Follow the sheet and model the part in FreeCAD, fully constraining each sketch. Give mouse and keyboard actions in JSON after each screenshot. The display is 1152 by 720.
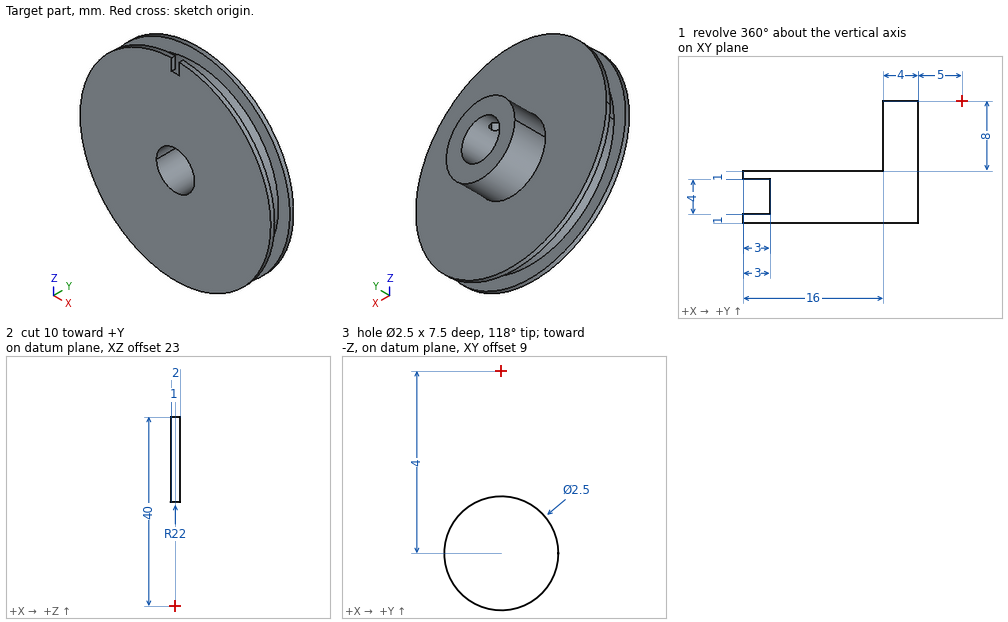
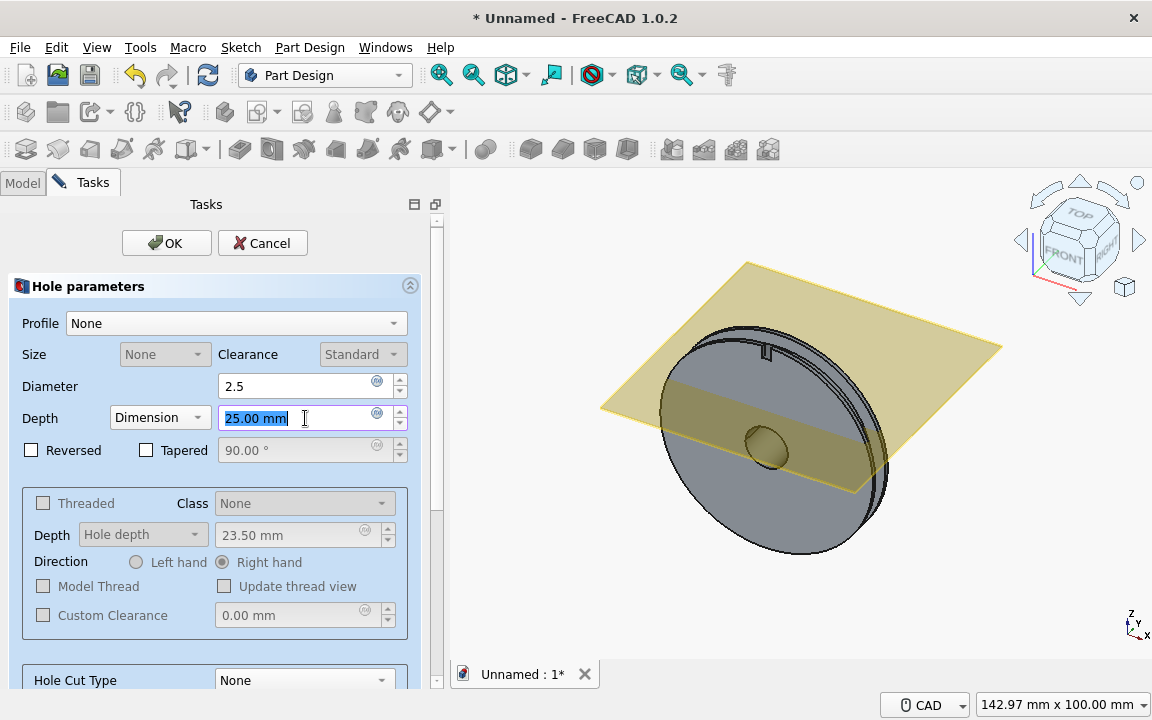
{"action": "type", "text": "7.5"}
{"action": "key", "text": "Tab"}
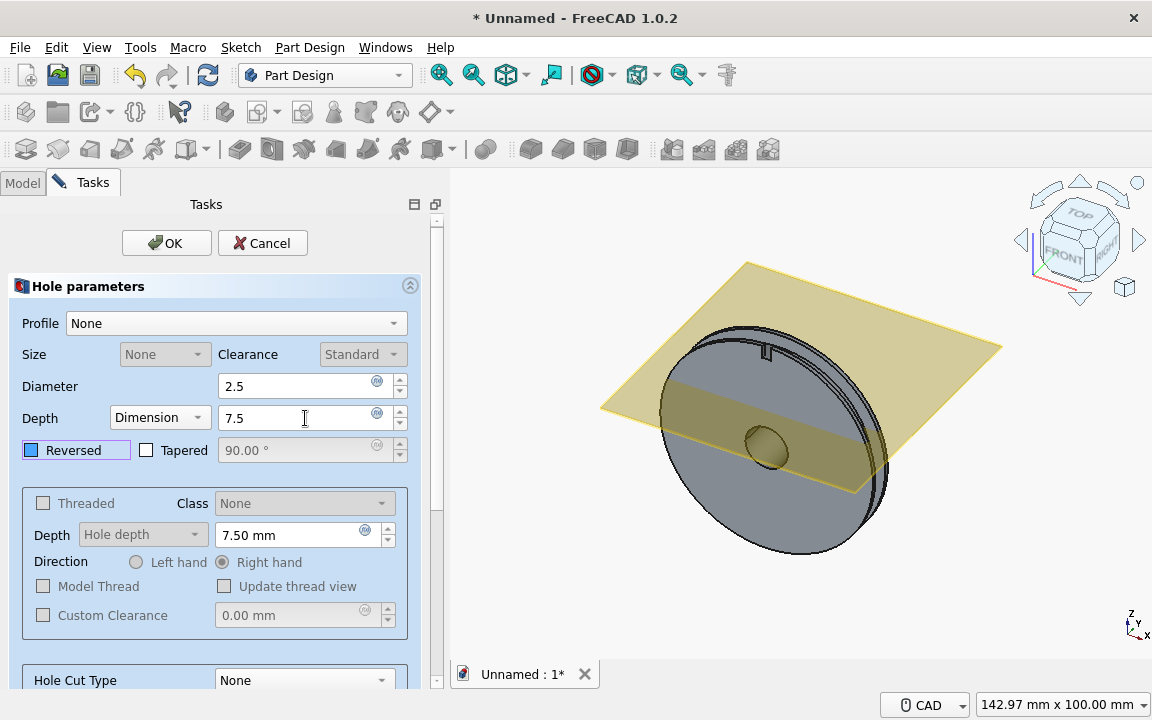
{"action": "left_click", "coordinate": [167, 243]}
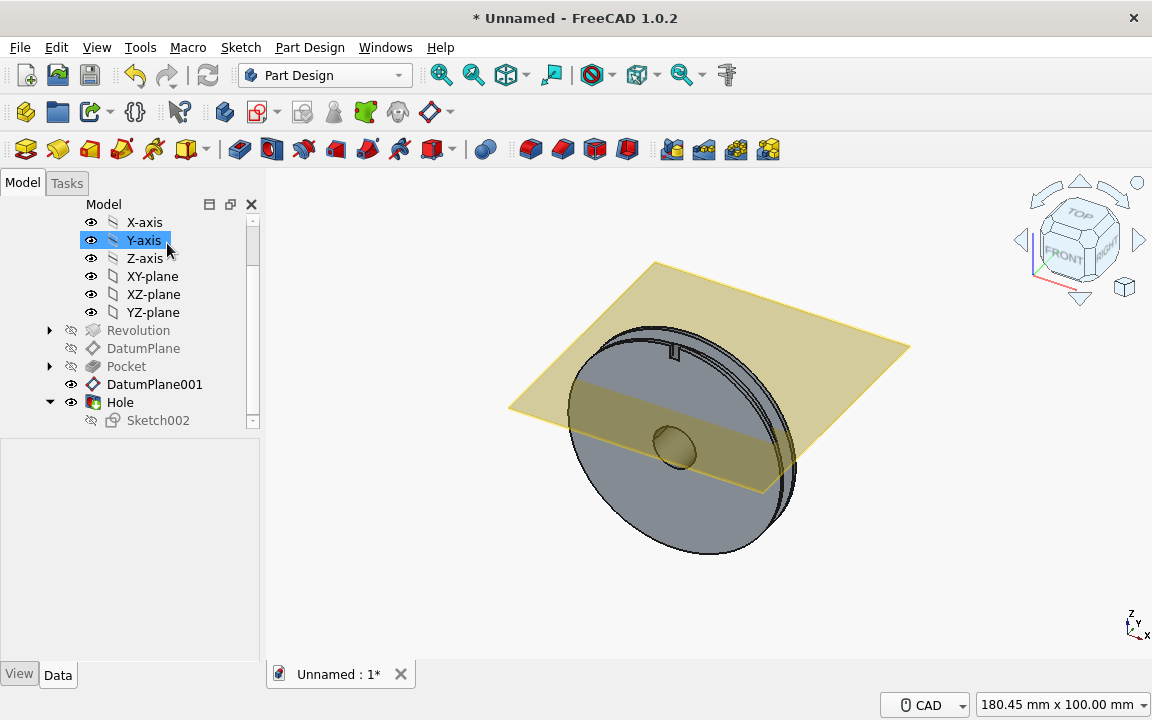
{"action": "left_click", "coordinate": [116, 384]}
{"action": "key", "text": "space"}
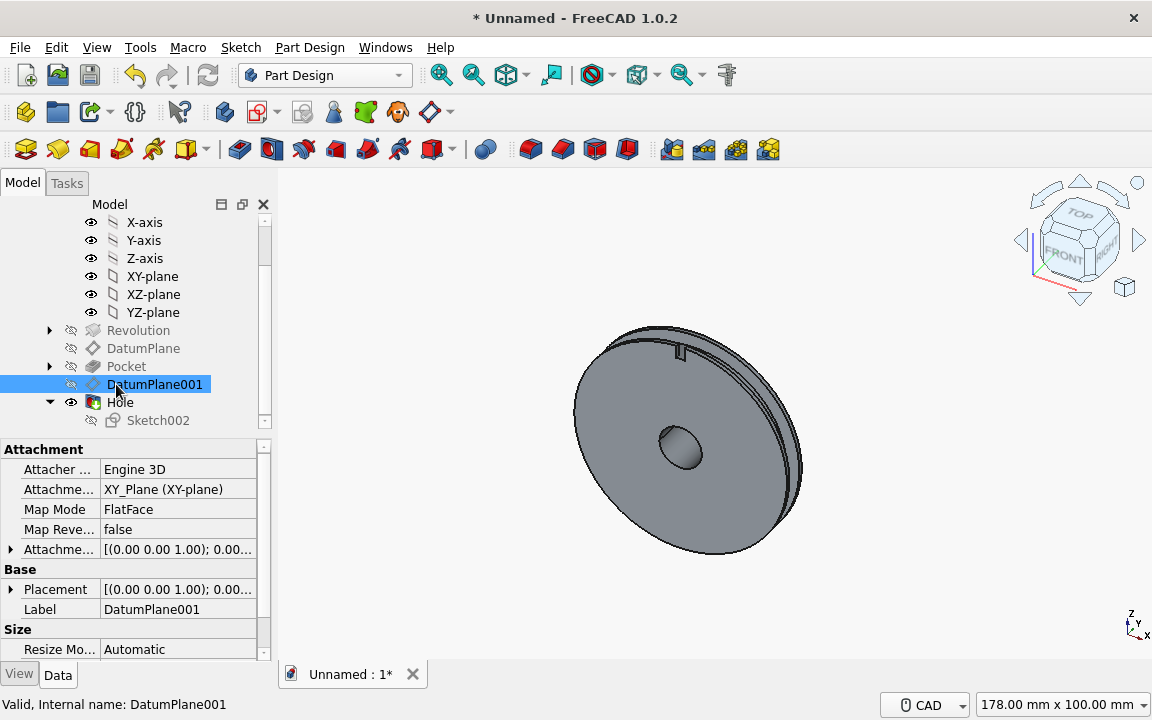
{"action": "key", "text": "0"}